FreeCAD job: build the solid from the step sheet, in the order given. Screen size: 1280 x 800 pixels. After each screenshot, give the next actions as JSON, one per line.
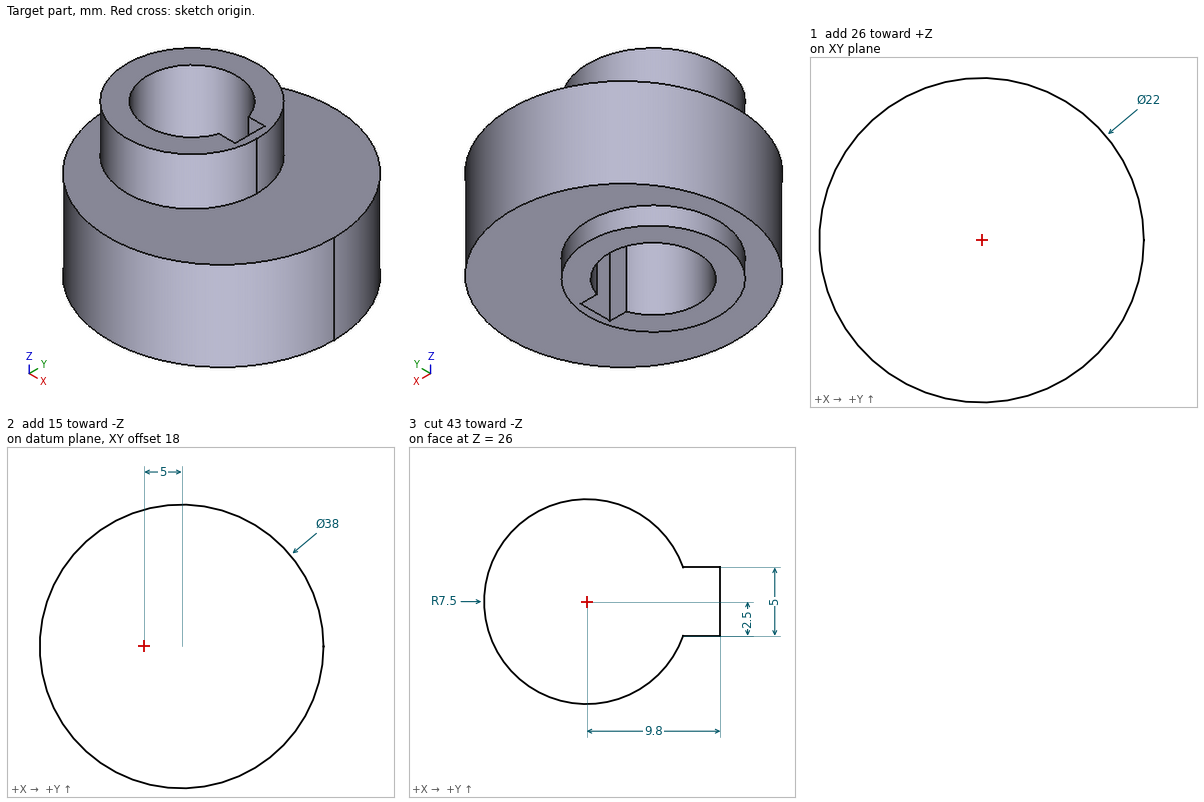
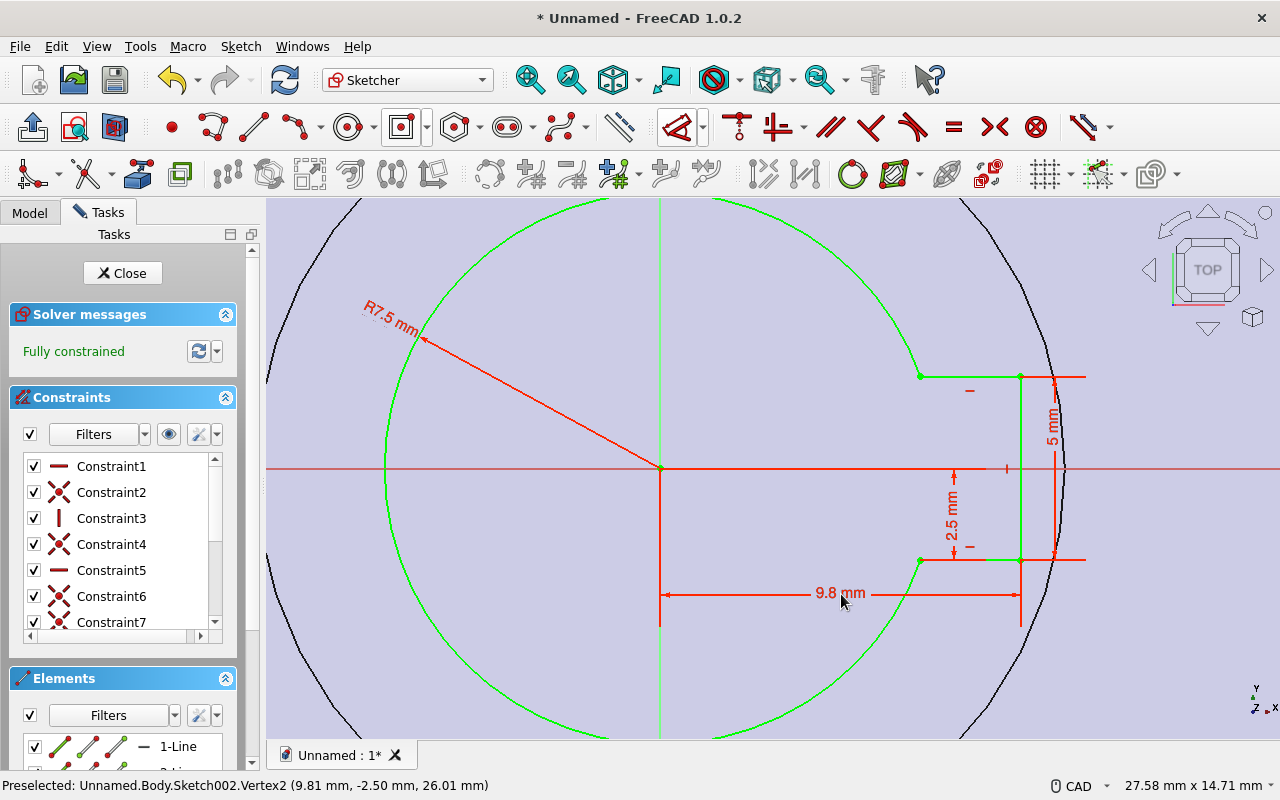
{"action": "left_click", "coordinate": [123, 273]}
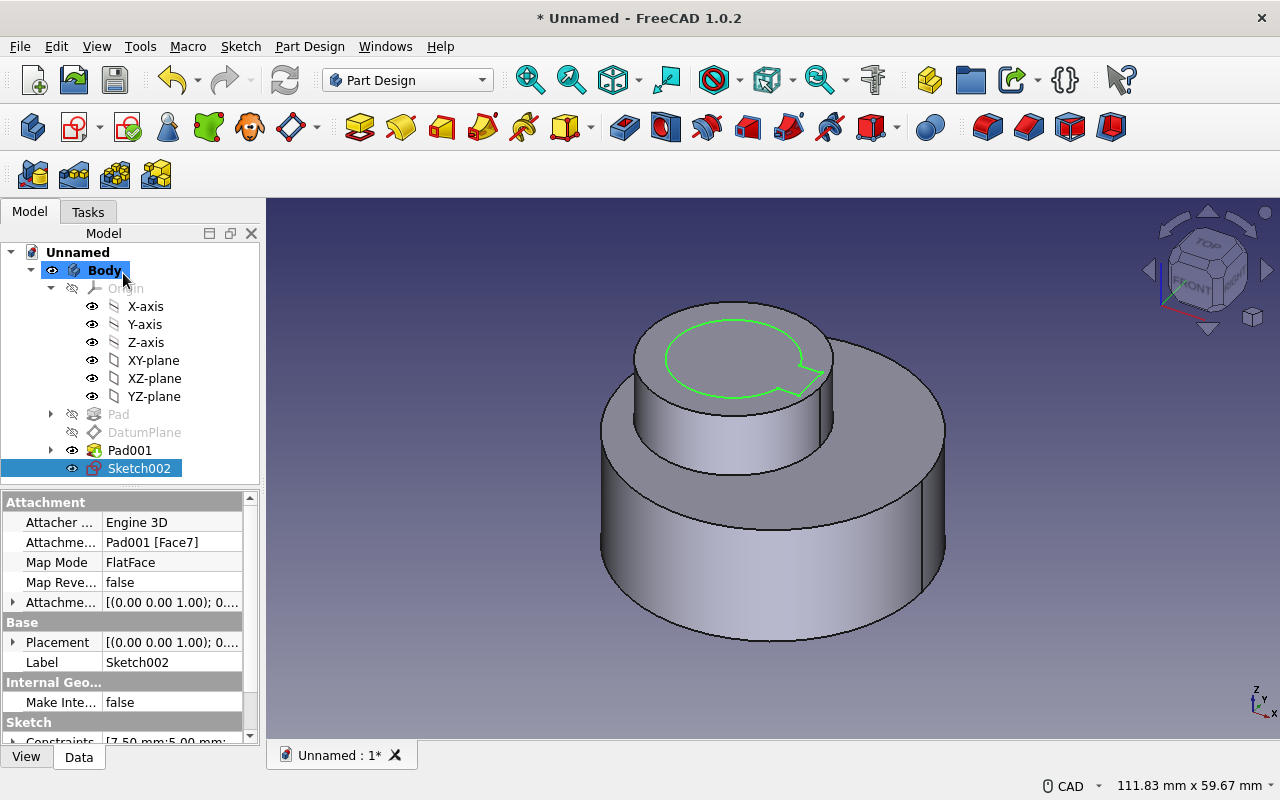
{"action": "left_click", "coordinate": [625, 128]}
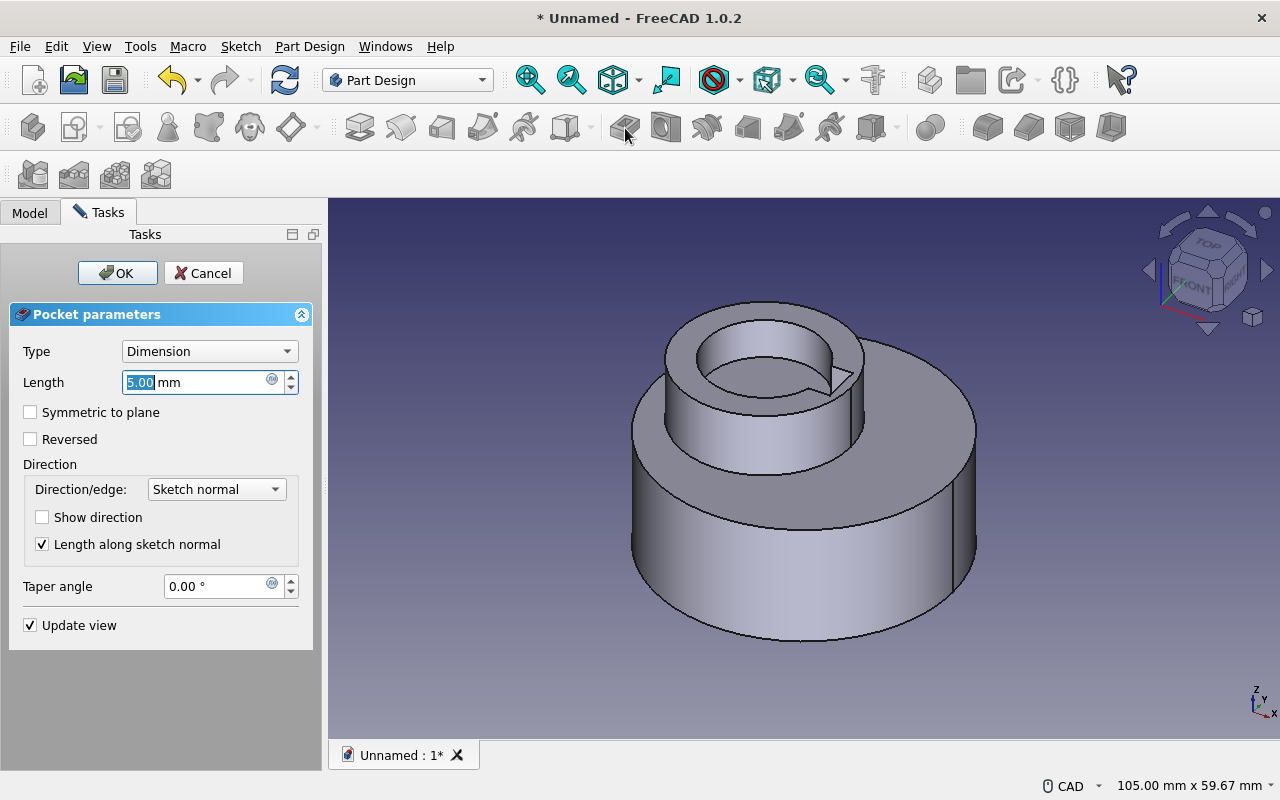
{"action": "type", "text": "43"}
{"action": "key", "text": "Tab"}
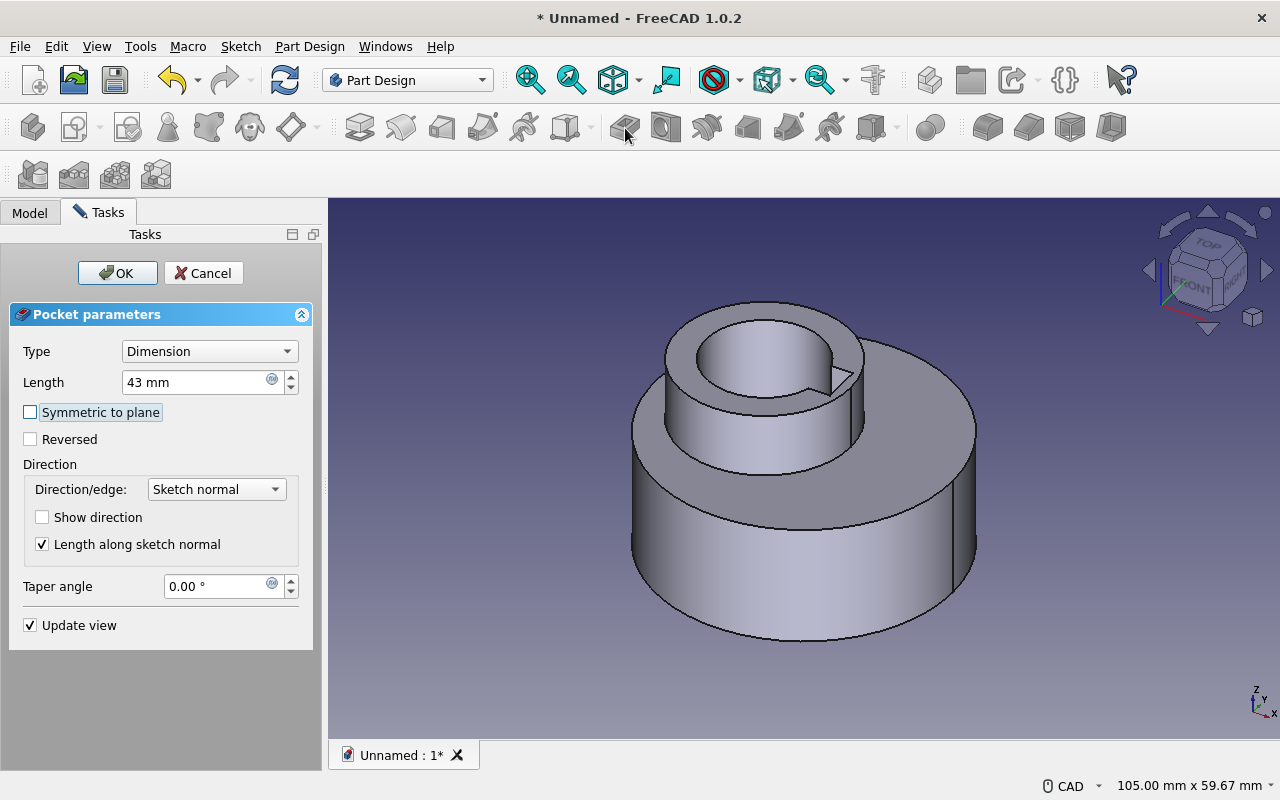
{"action": "left_click", "coordinate": [118, 273]}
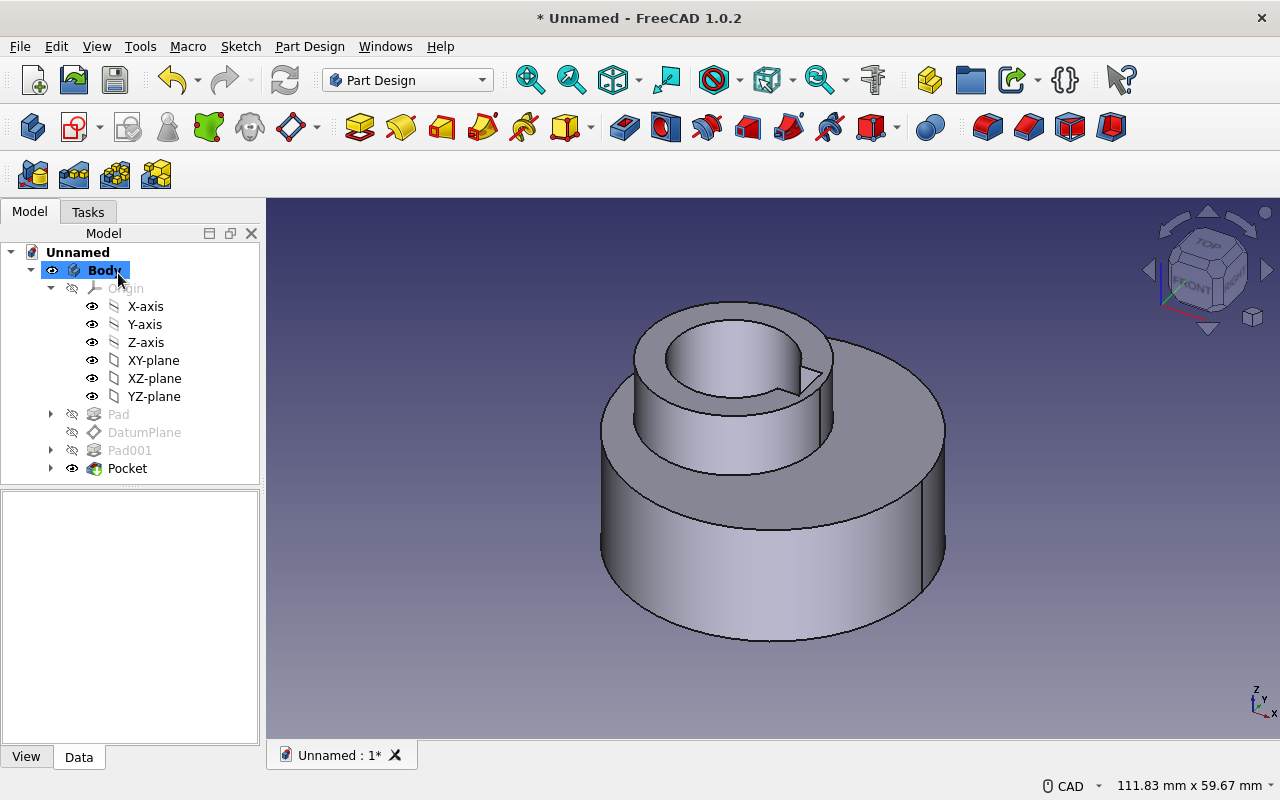
{"action": "key", "text": "0"}